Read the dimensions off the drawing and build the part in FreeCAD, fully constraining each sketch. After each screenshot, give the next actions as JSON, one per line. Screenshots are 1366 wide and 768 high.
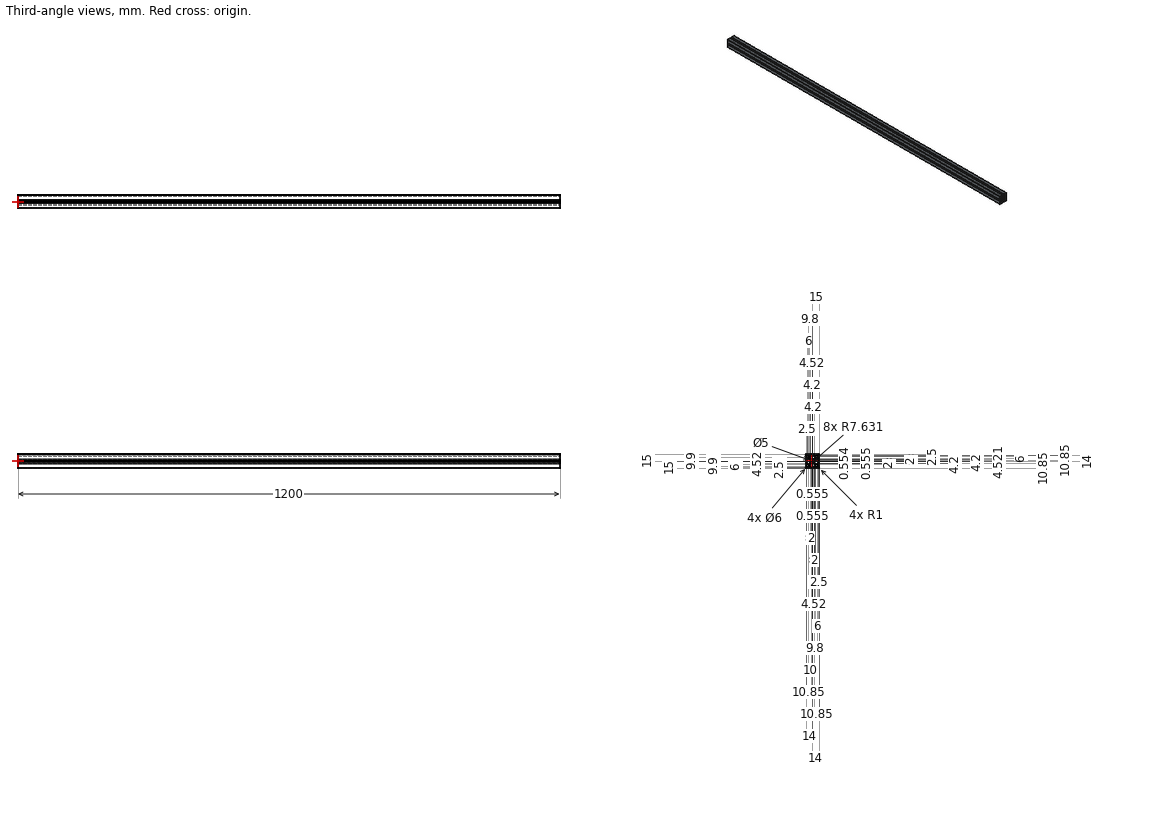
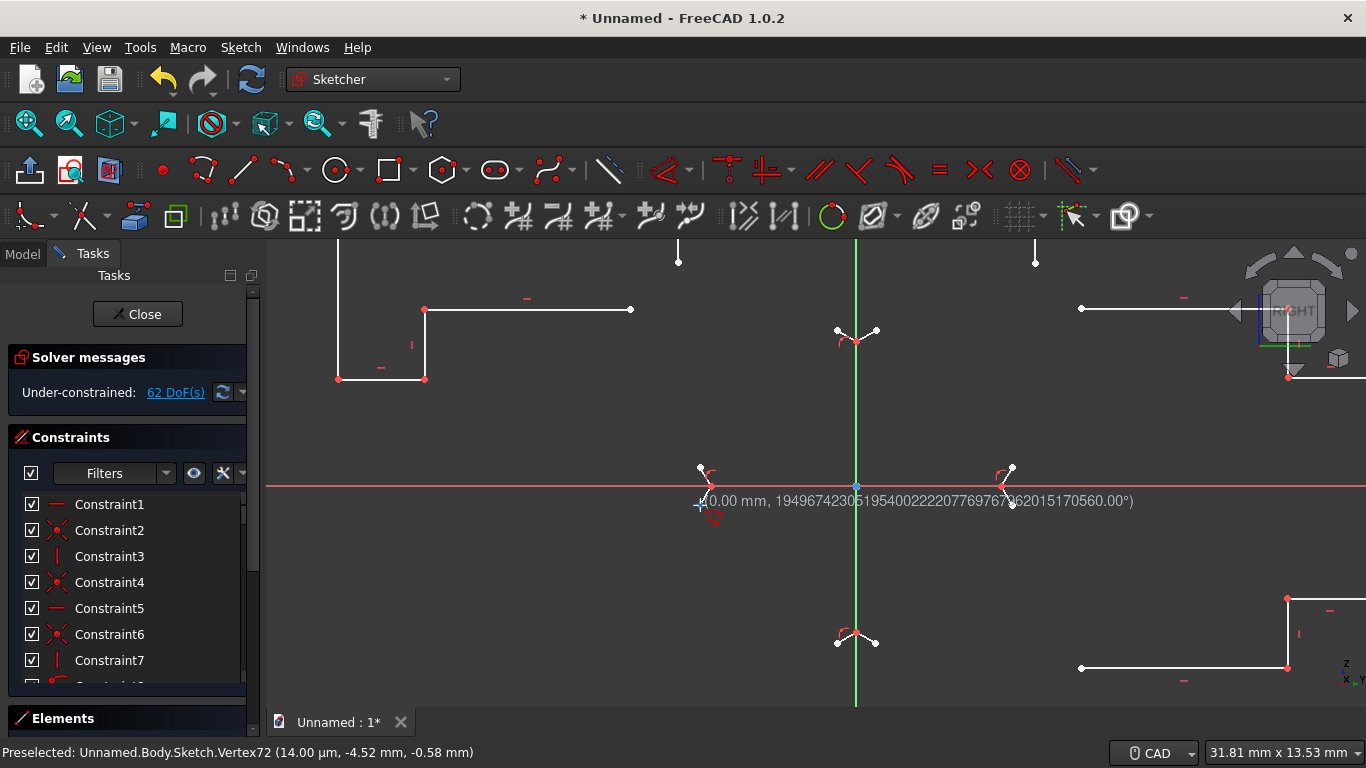
{"action": "left_click", "coordinate": [632, 664]}
{"action": "left_click", "coordinate": [424, 664]}
{"action": "left_click", "coordinate": [424, 595]}
{"action": "left_click", "coordinate": [338, 595]}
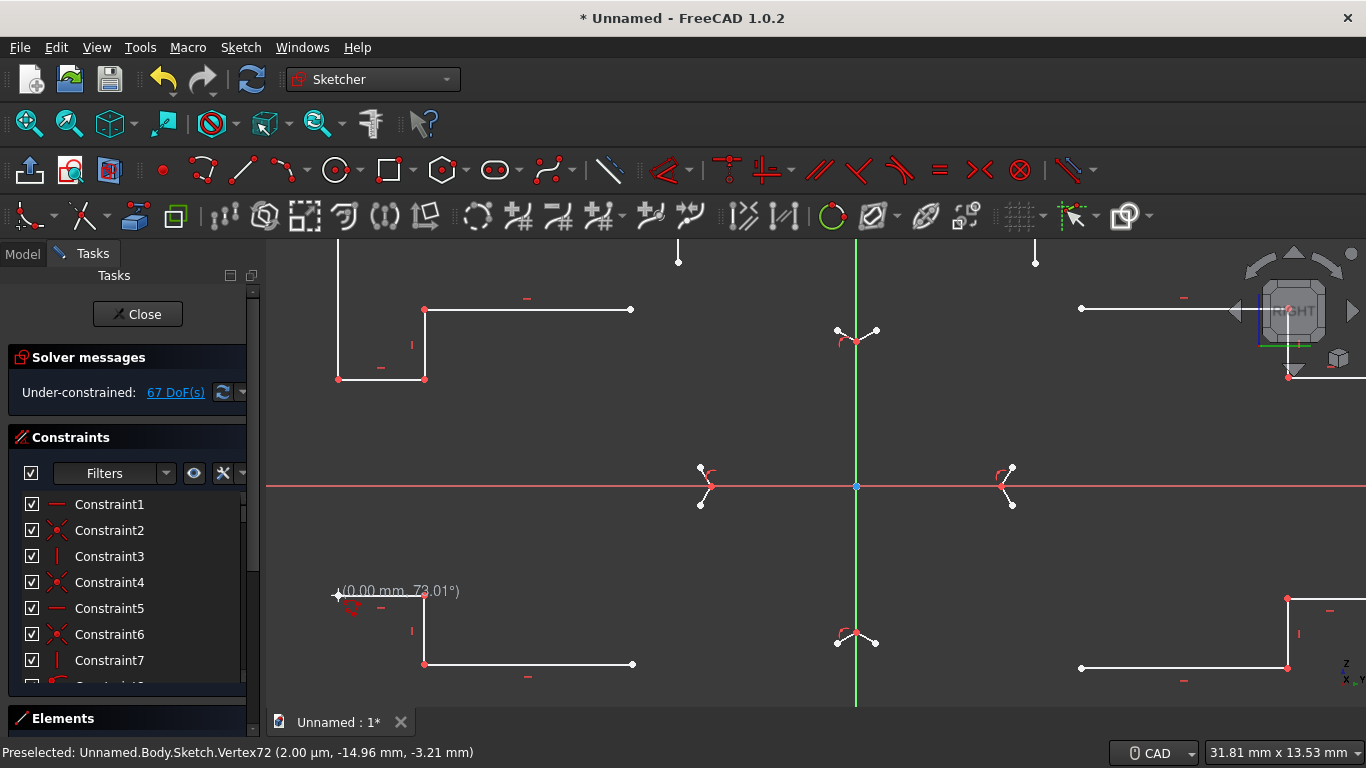
{"action": "scroll", "coordinate": [701, 467], "scroll_direction": "down", "scroll_amount": 6}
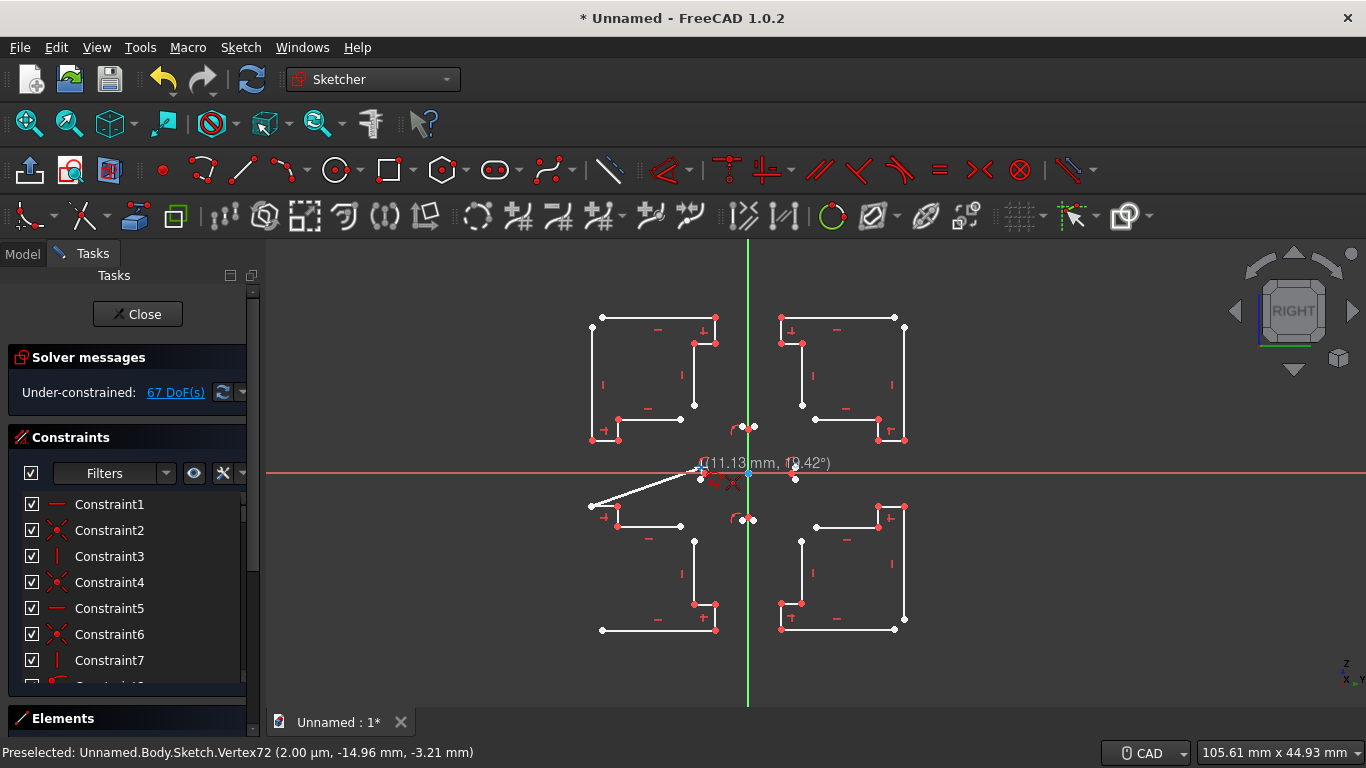
{"action": "left_click", "coordinate": [592, 619]}
{"action": "right_click", "coordinate": [592, 619]}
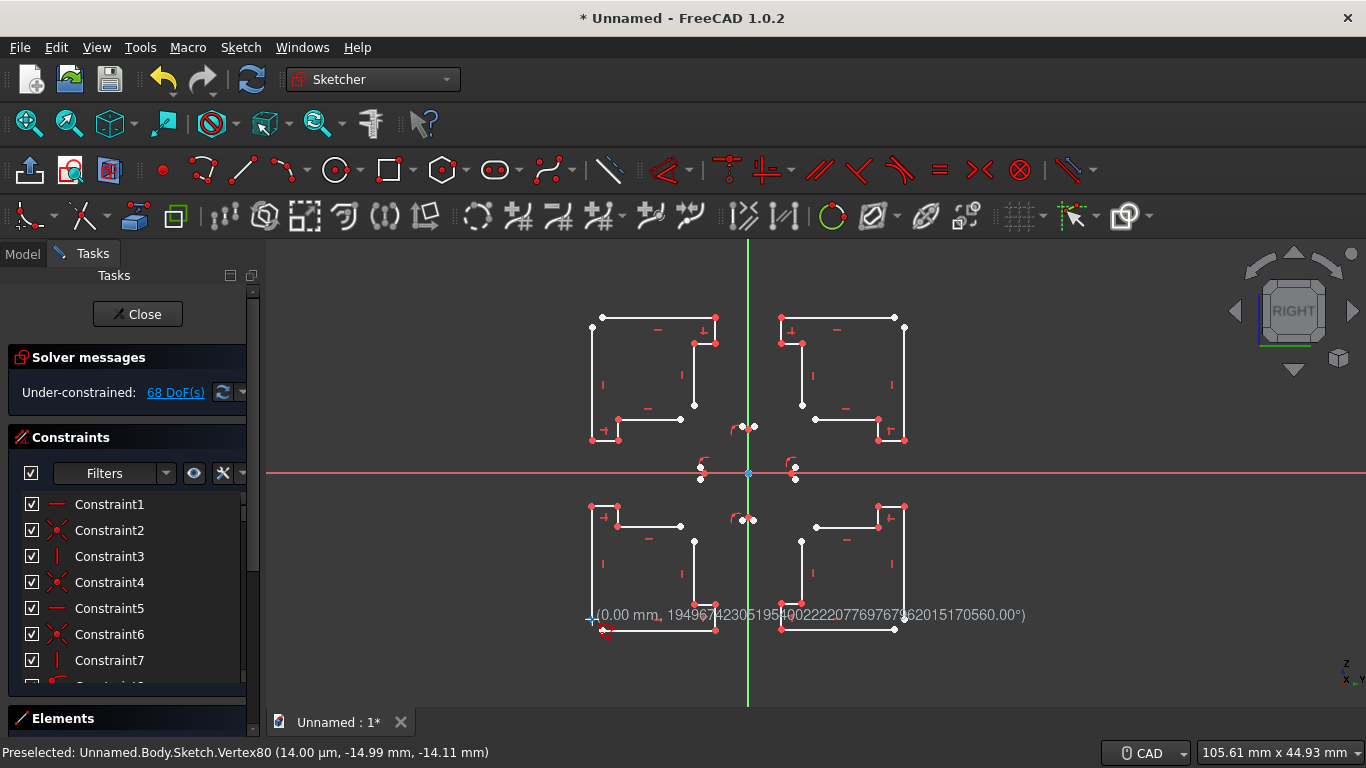
{"action": "left_click", "coordinate": [284, 170]}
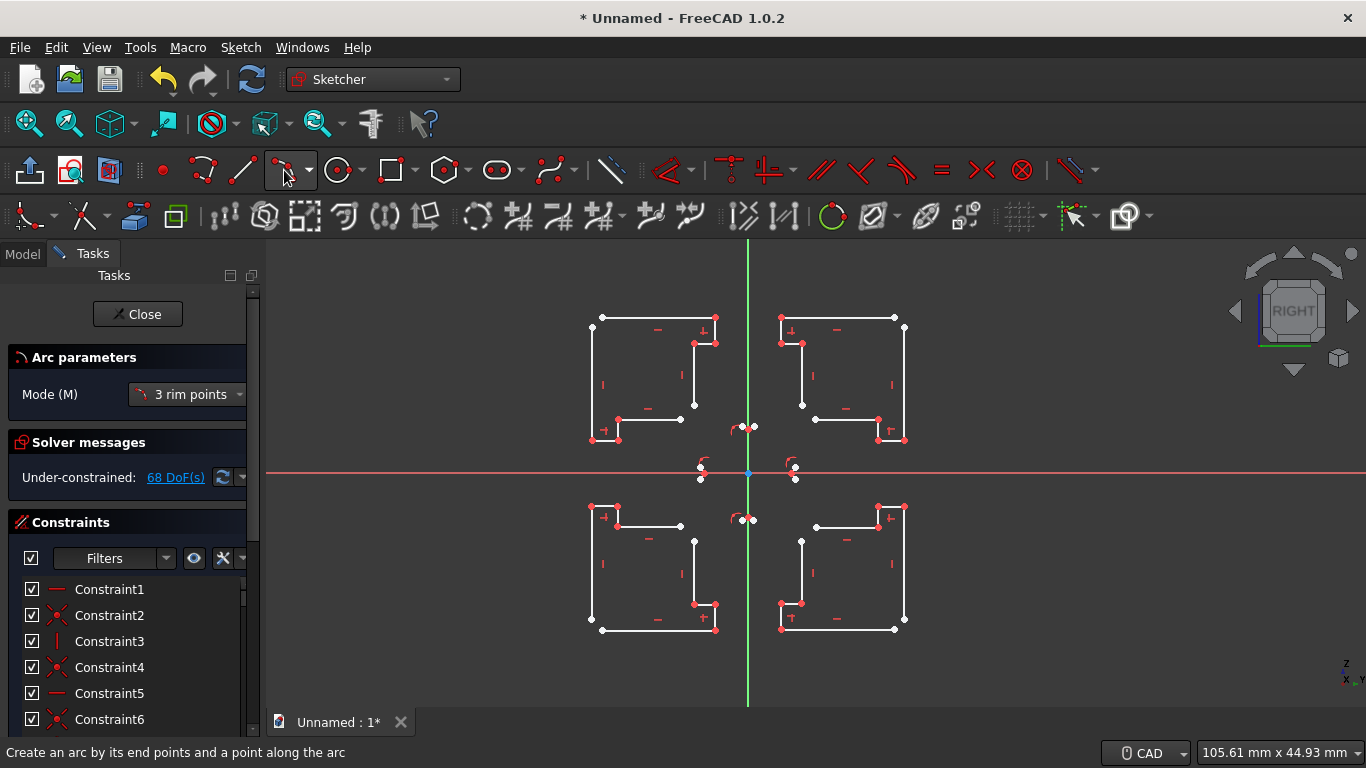
{"action": "left_click", "coordinate": [694, 542]}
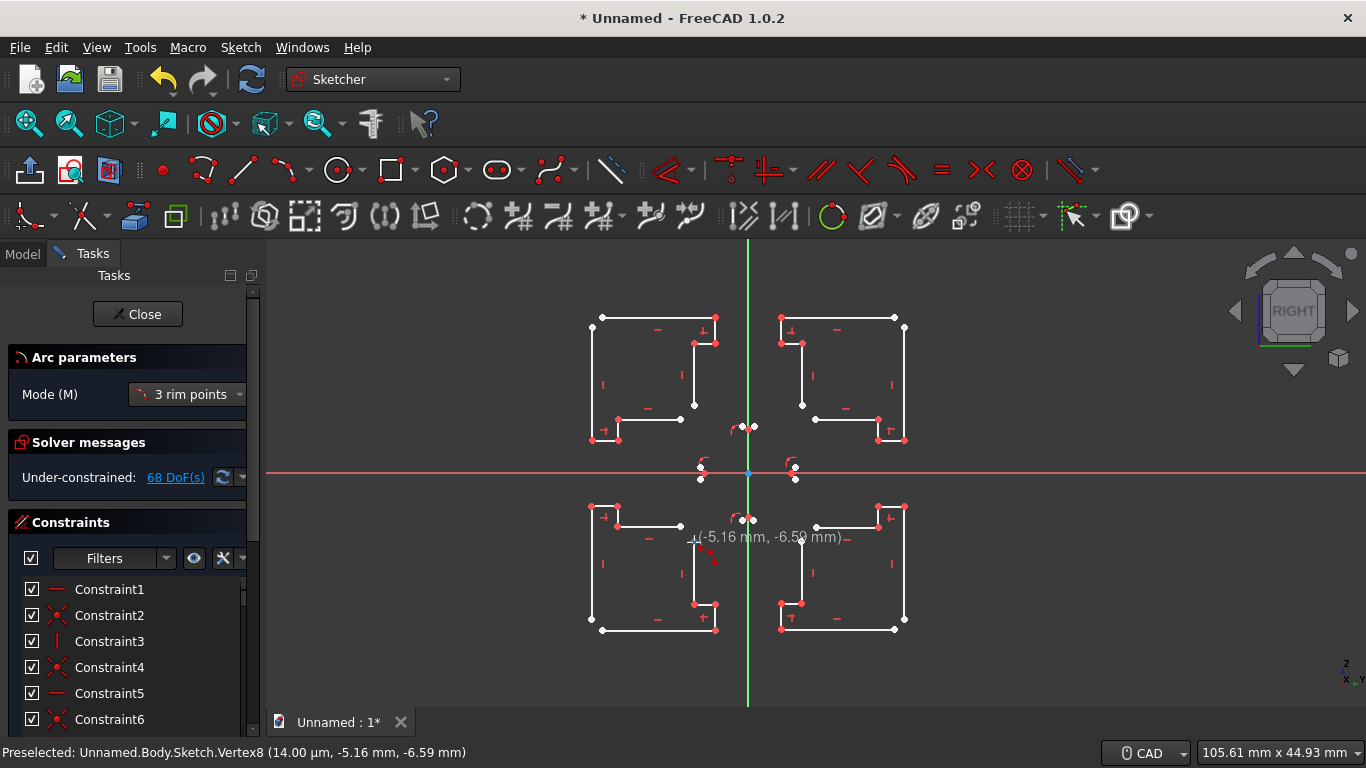
{"action": "scroll", "coordinate": [742, 520], "scroll_direction": "up", "scroll_amount": 8}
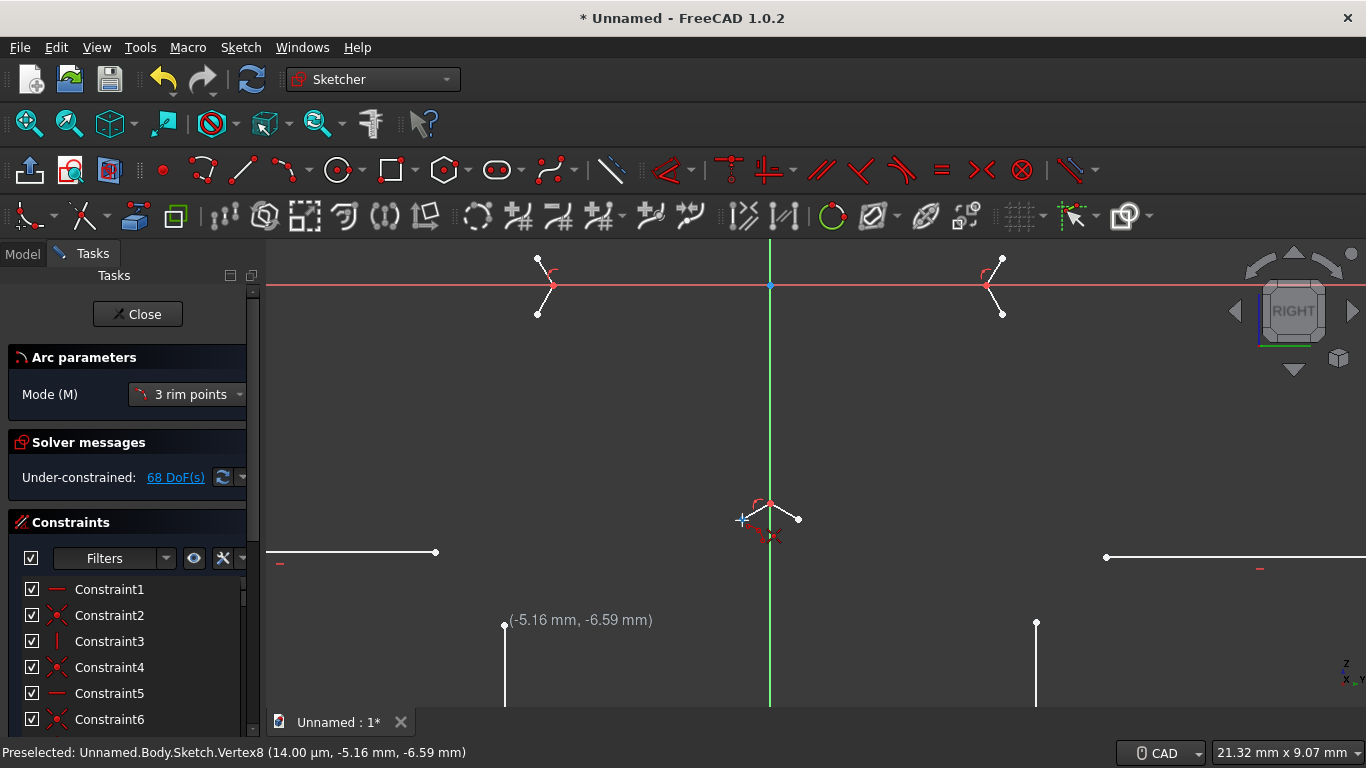
{"action": "left_click", "coordinate": [742, 520]}
{"action": "left_click", "coordinate": [615, 550]}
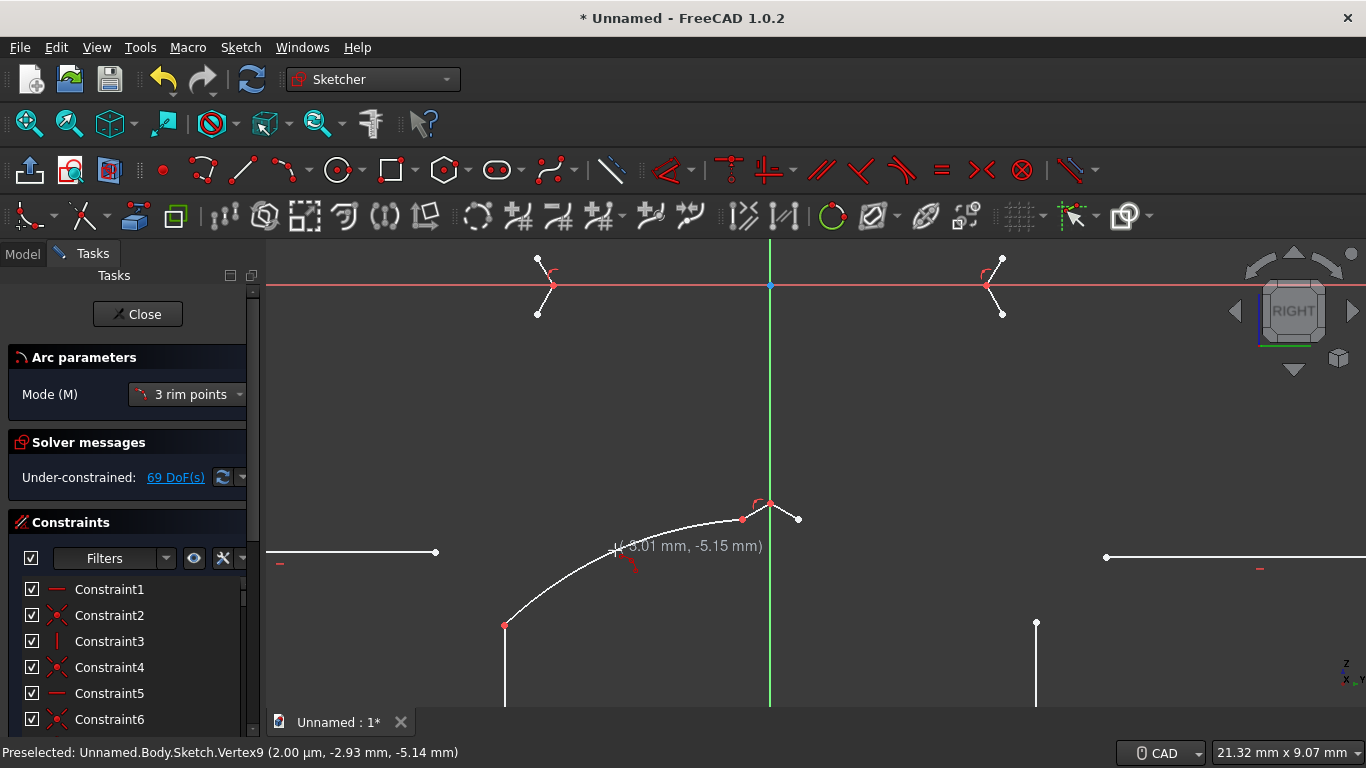
{"action": "left_click", "coordinate": [799, 520]}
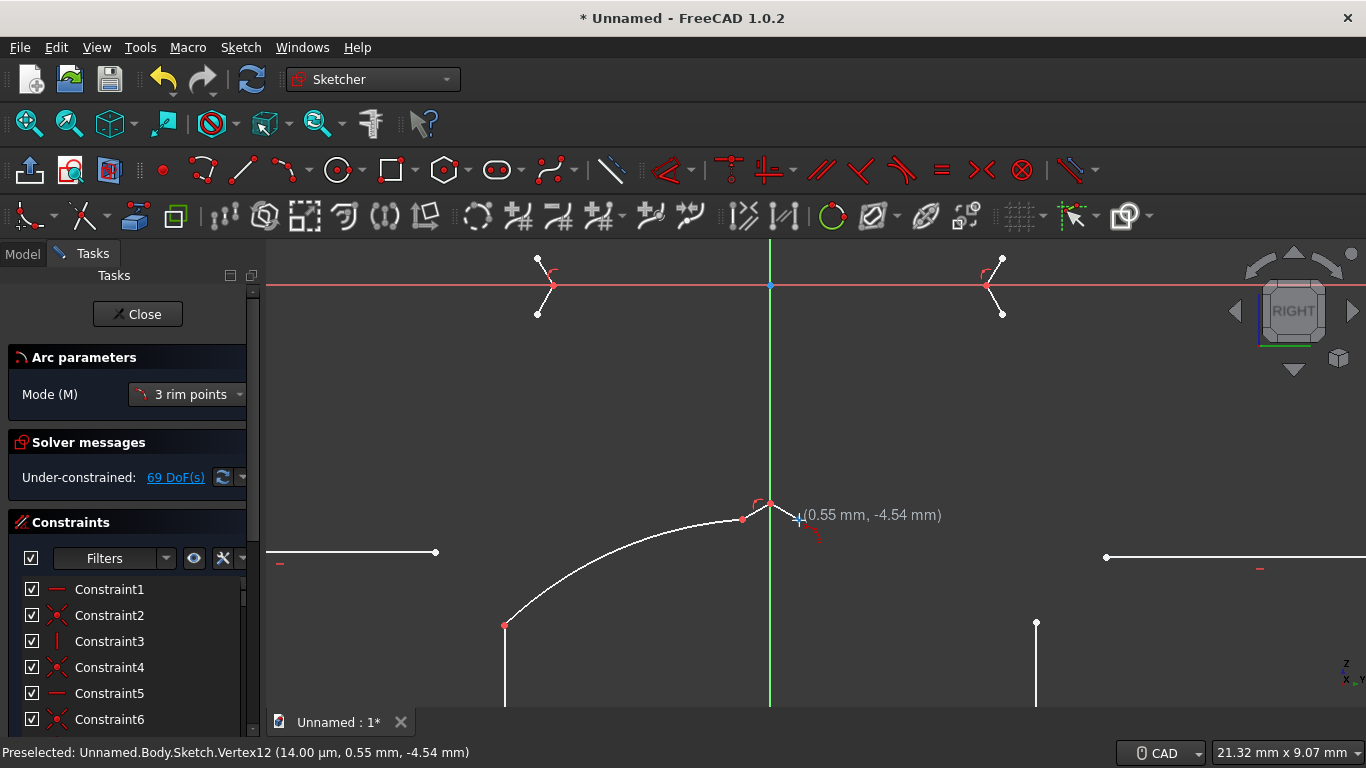
{"action": "scroll", "coordinate": [742, 520], "scroll_direction": "down", "scroll_amount": 8}